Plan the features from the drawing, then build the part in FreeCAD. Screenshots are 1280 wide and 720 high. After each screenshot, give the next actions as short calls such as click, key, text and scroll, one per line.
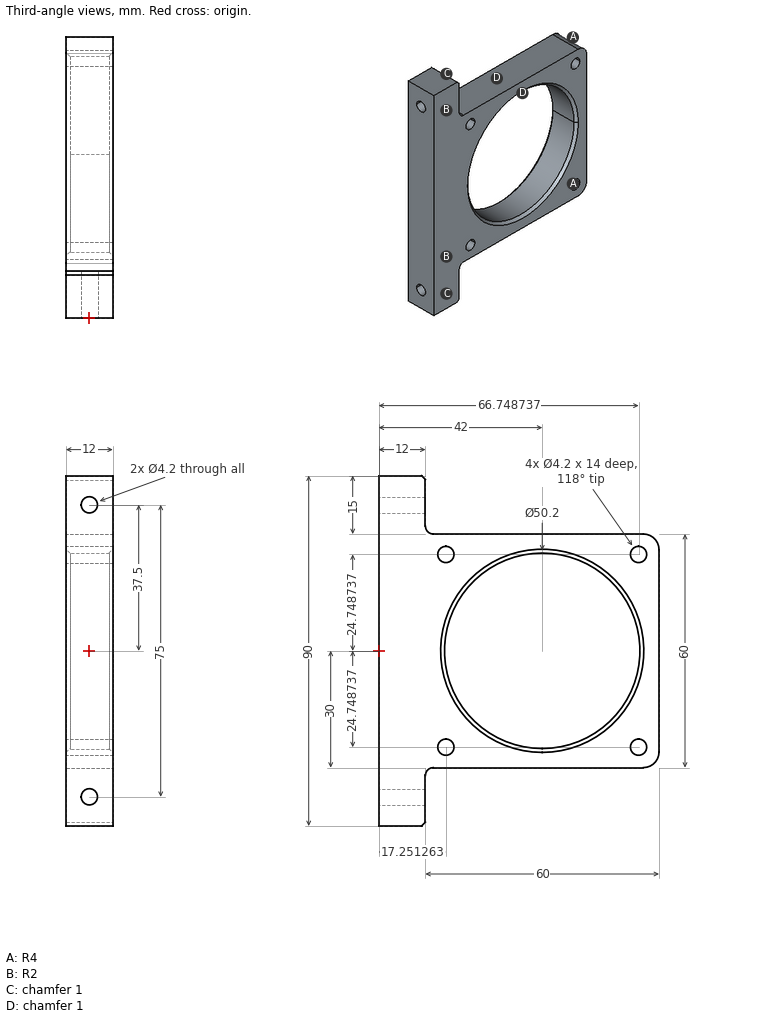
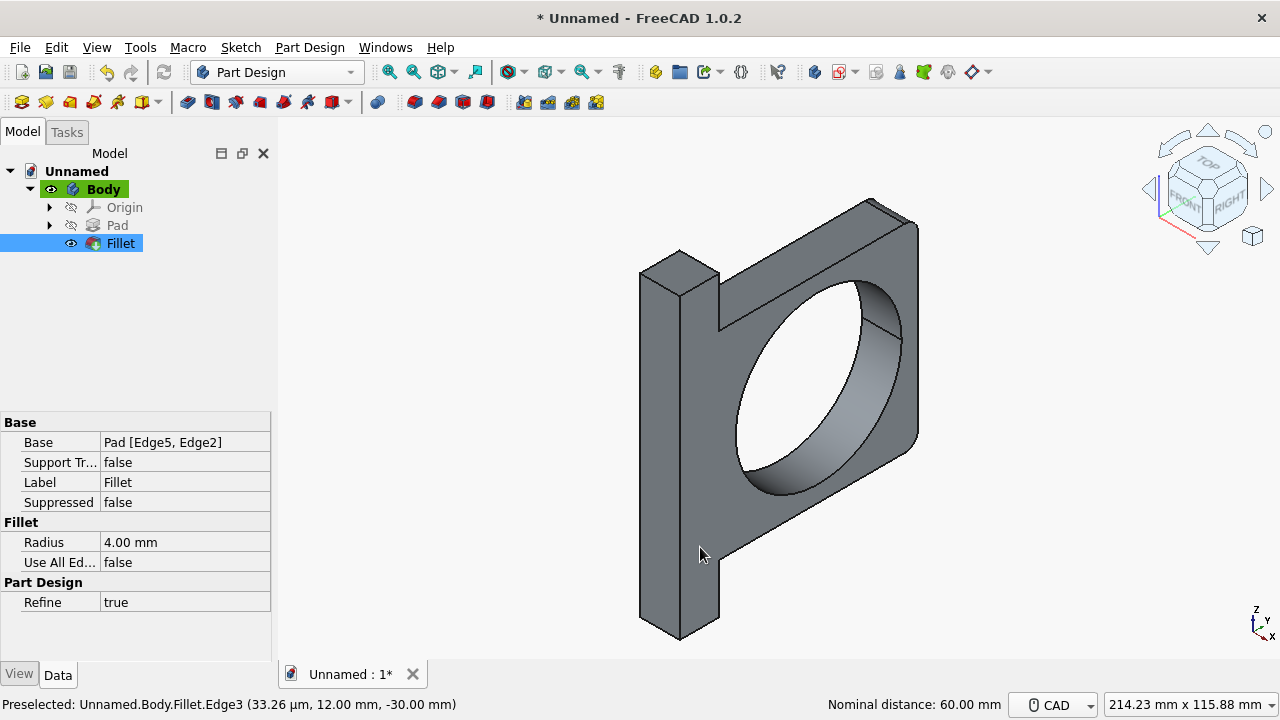
click(416, 102)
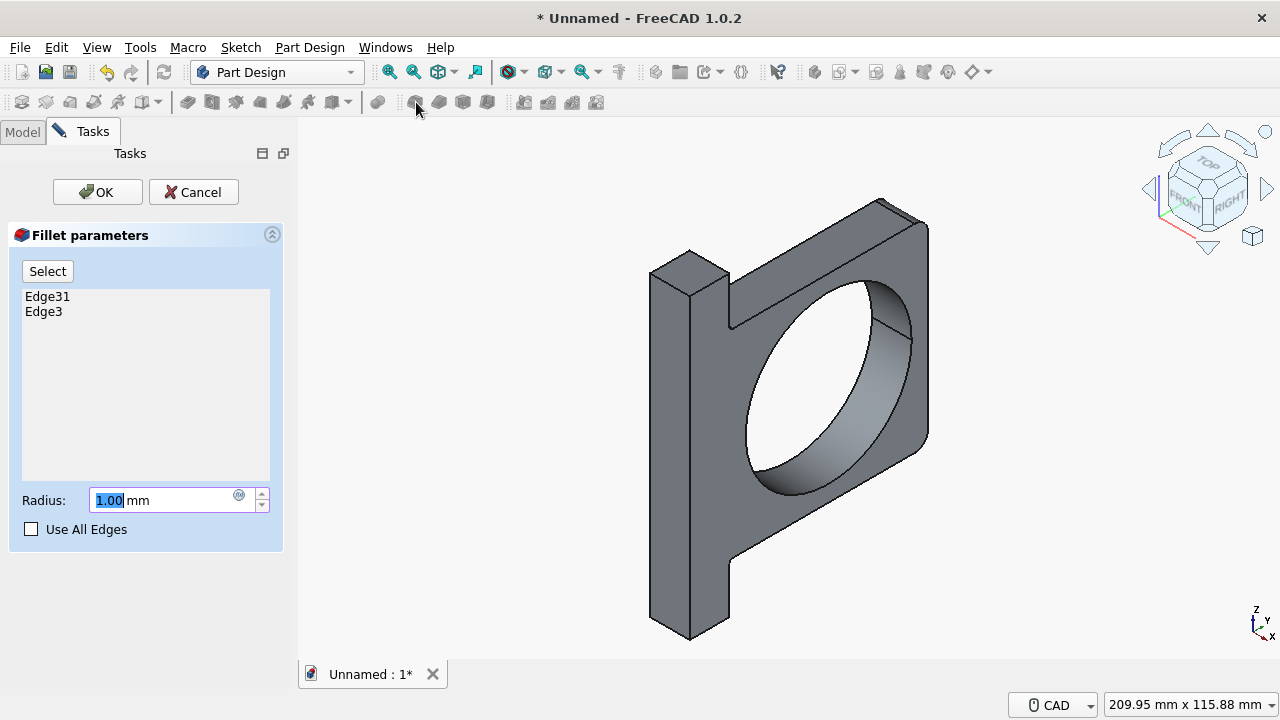
text(2)
key(Tab)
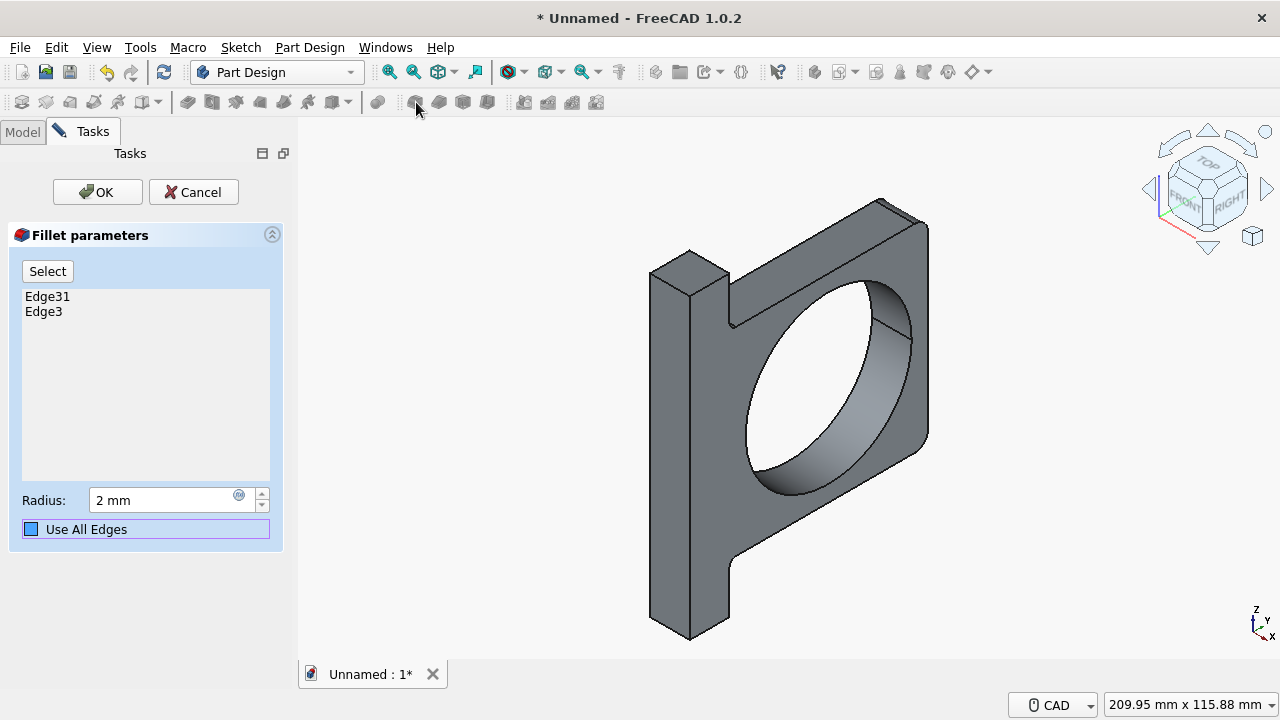
click(98, 192)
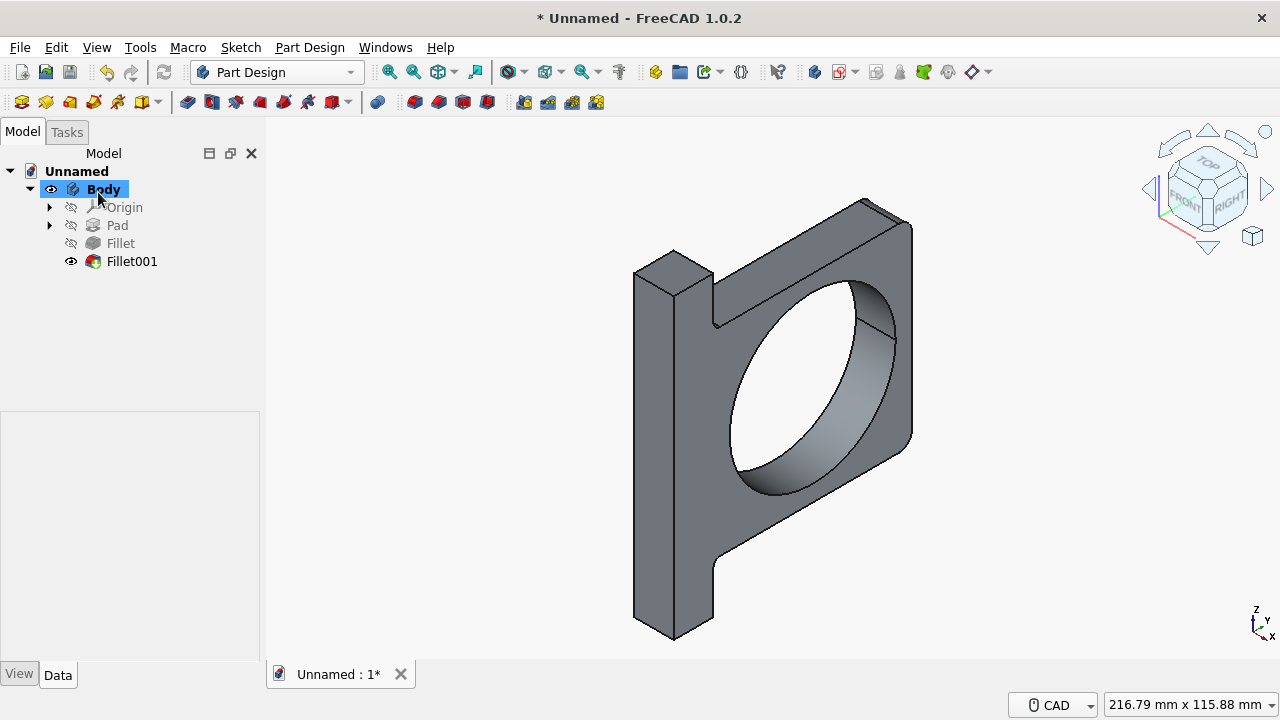
key(2)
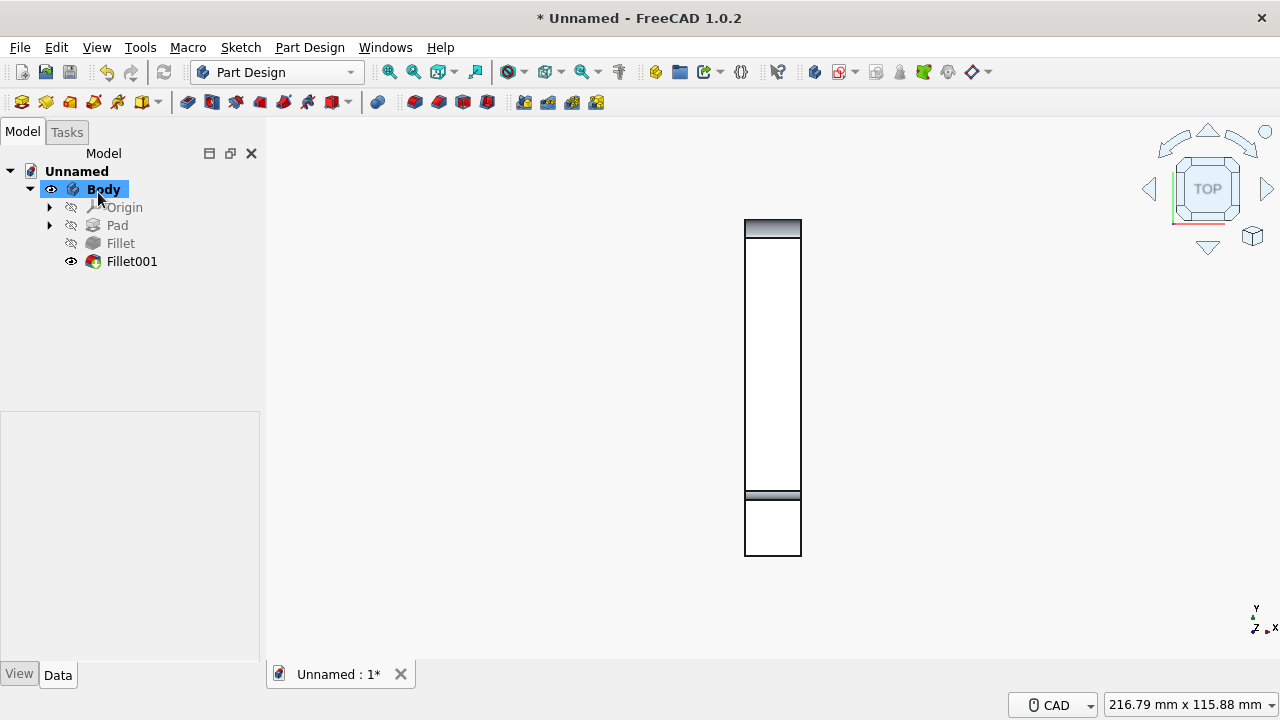
click(773, 499)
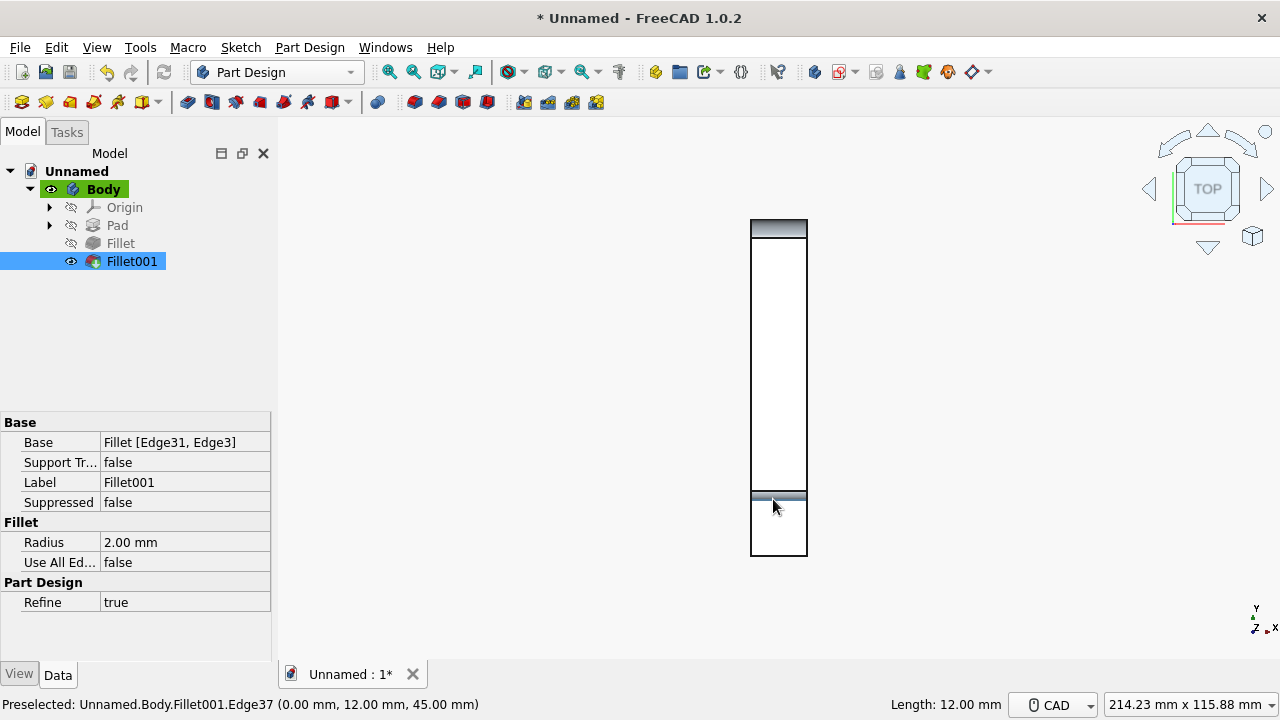
key(0)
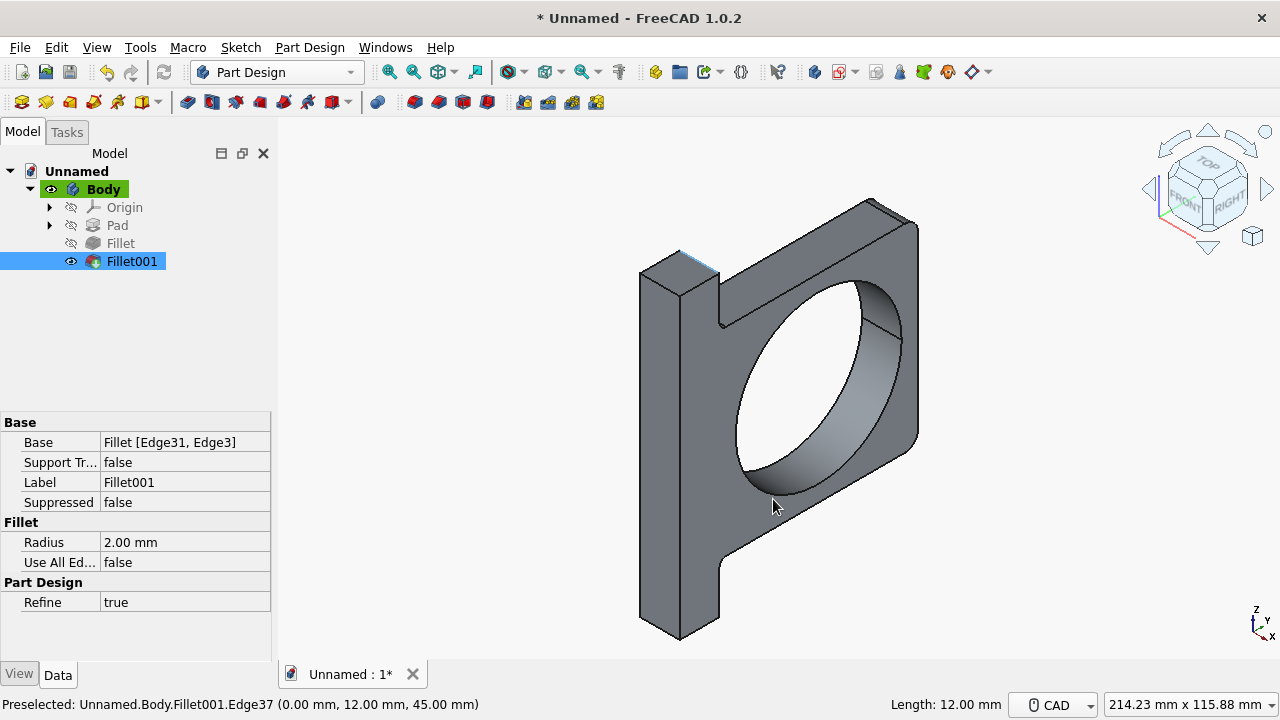
key(1)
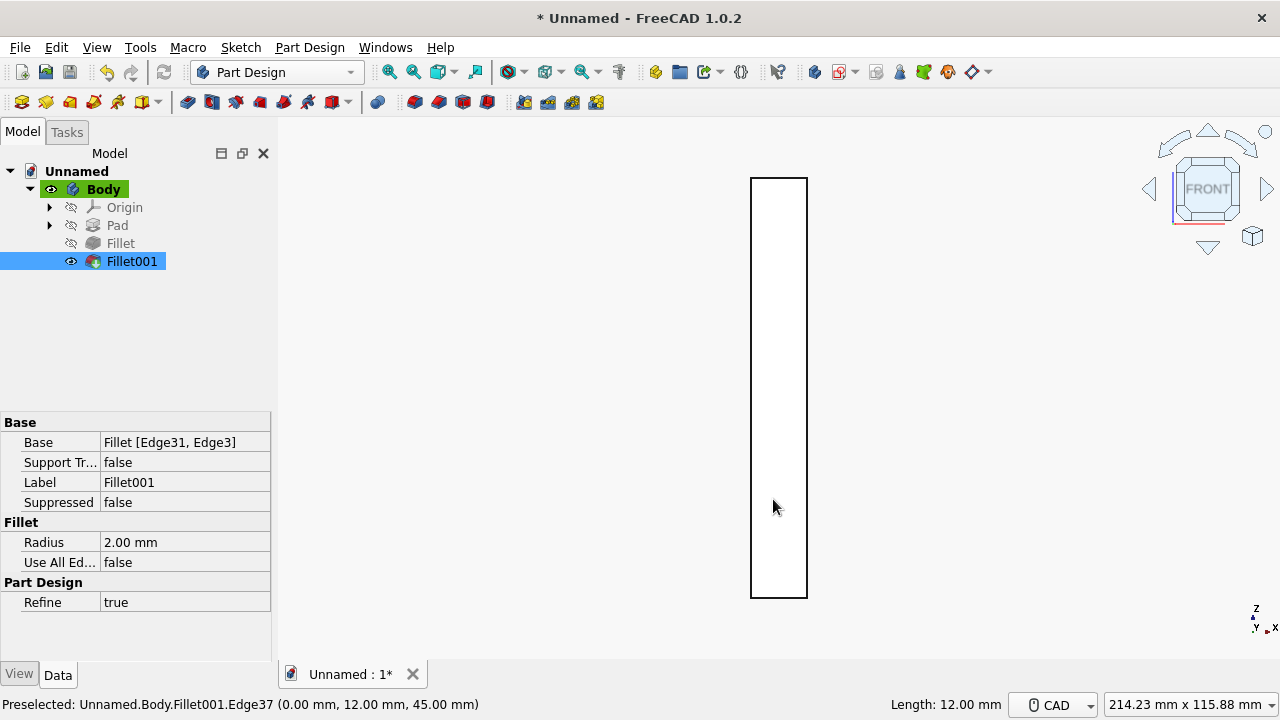
key(3)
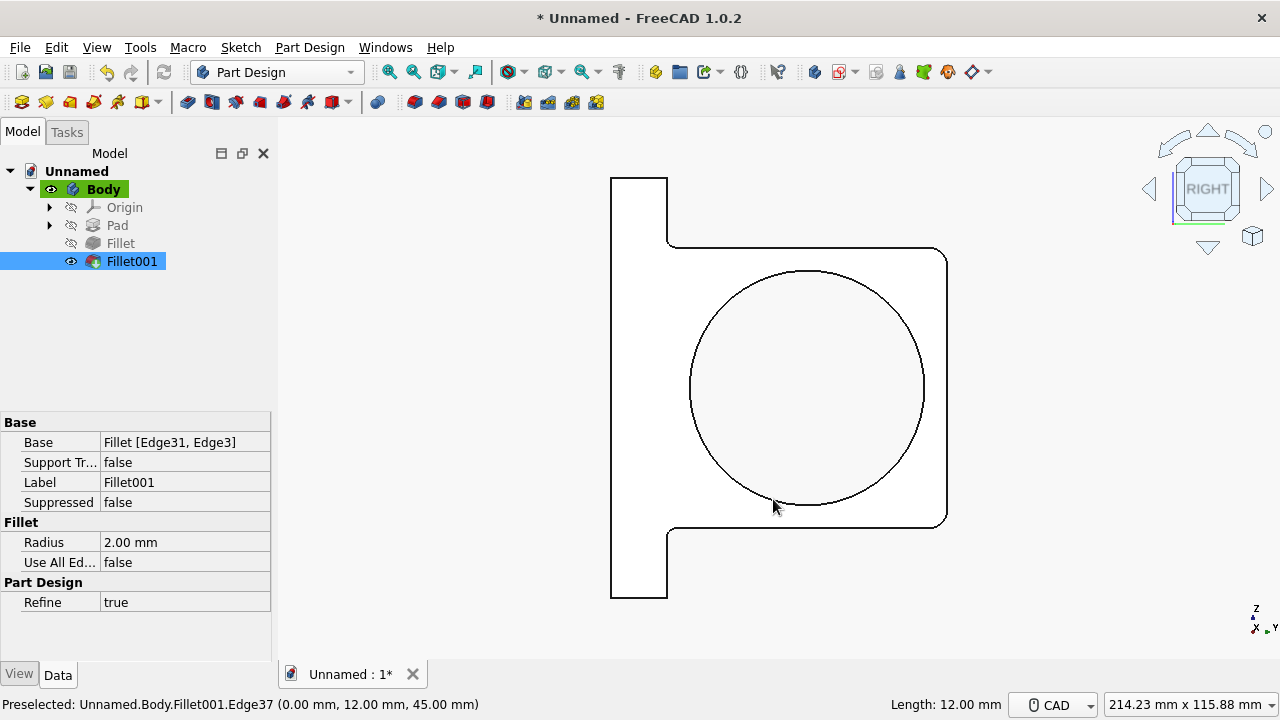
key(5)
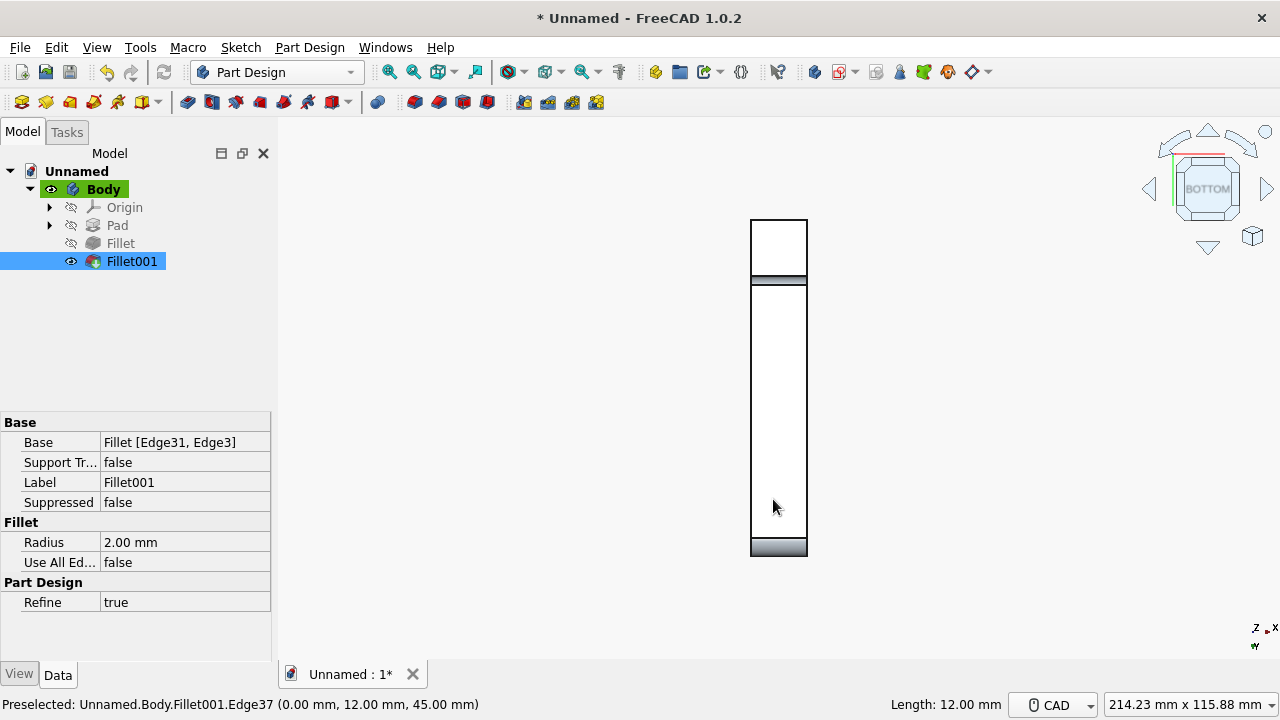
click(779, 275, ctrl)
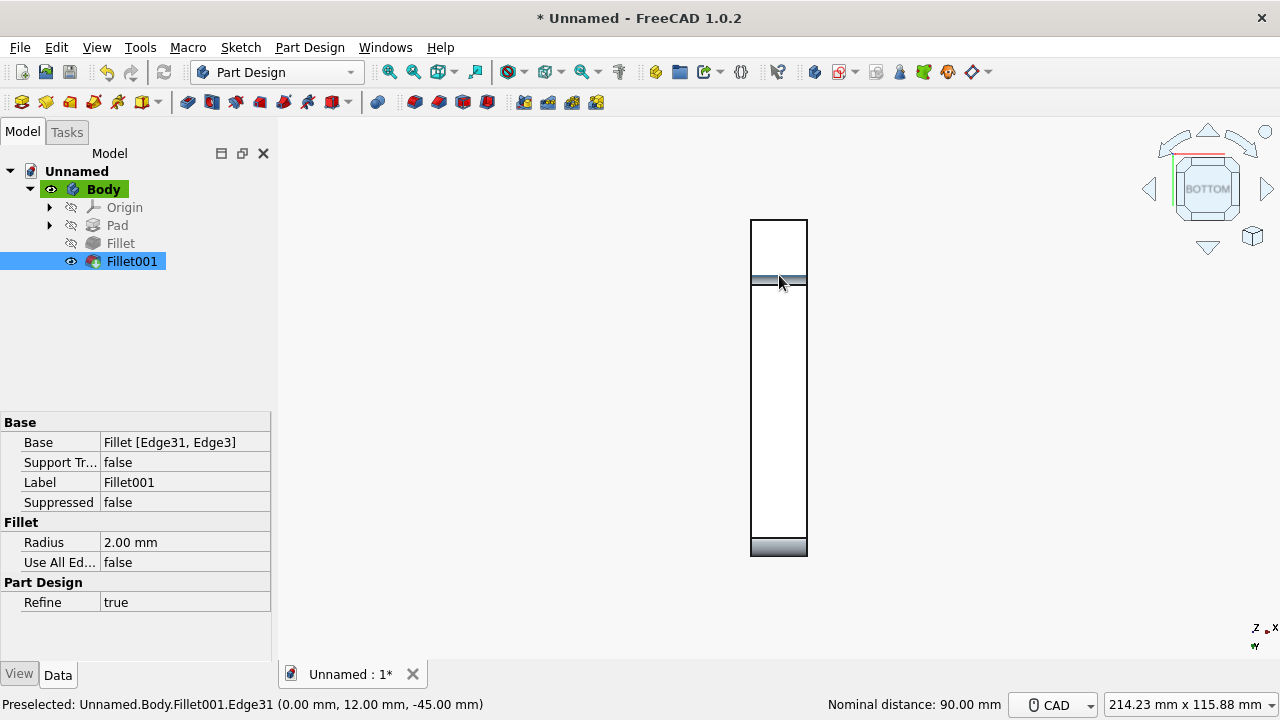
click(440, 102)